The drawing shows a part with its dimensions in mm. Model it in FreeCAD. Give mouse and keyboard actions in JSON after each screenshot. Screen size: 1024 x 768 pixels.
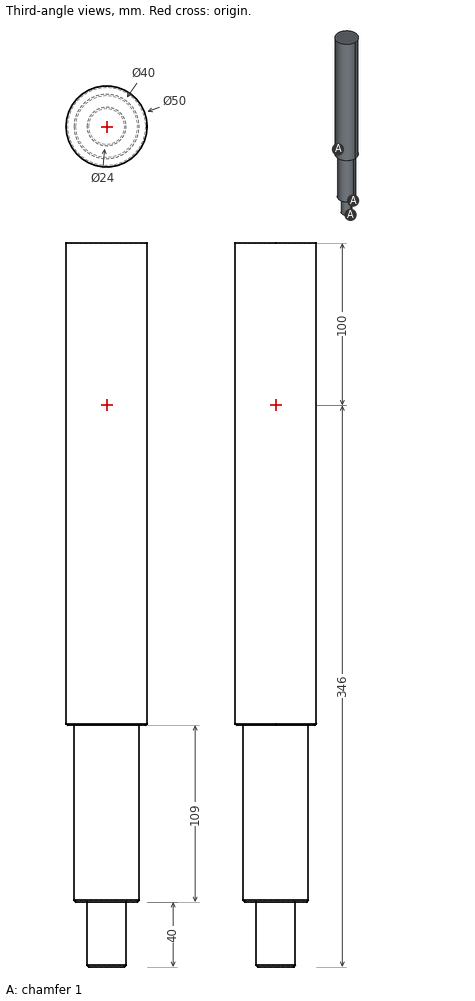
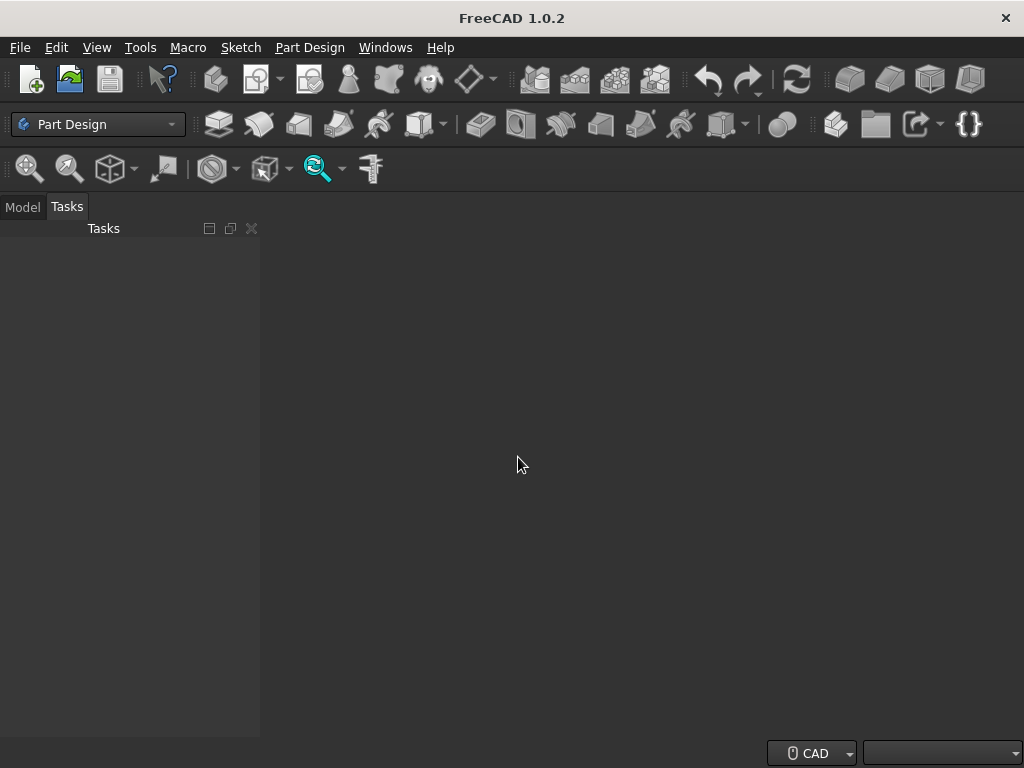
{"action": "left_click", "coordinate": [30, 80]}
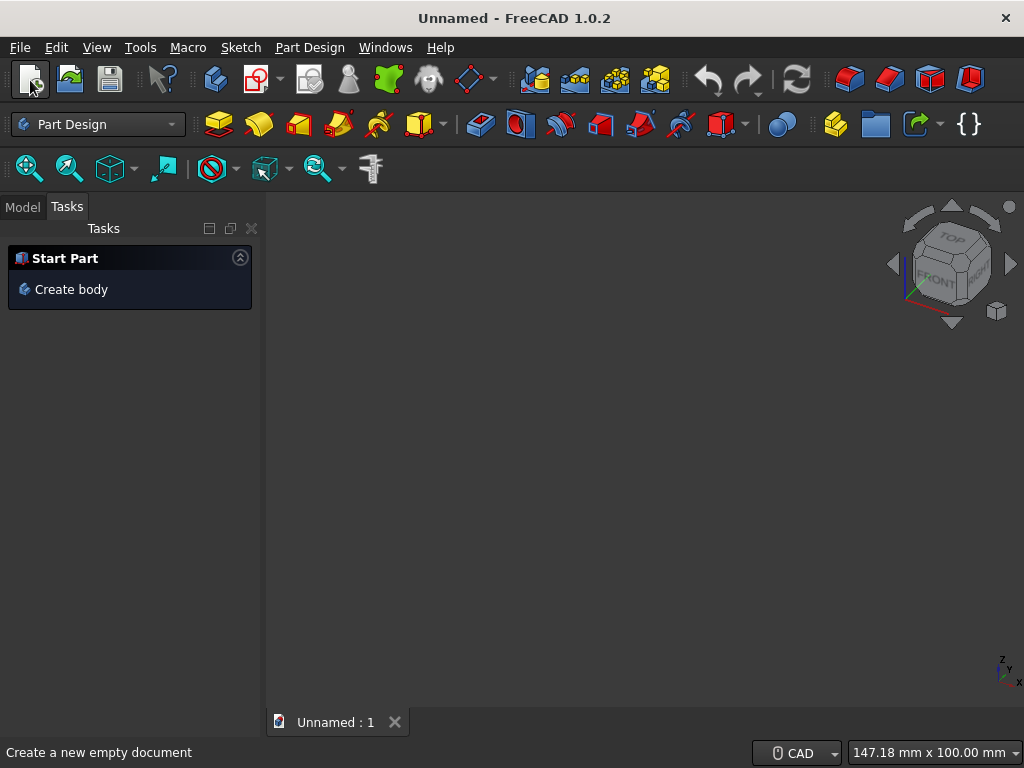
{"action": "left_click", "coordinate": [256, 80]}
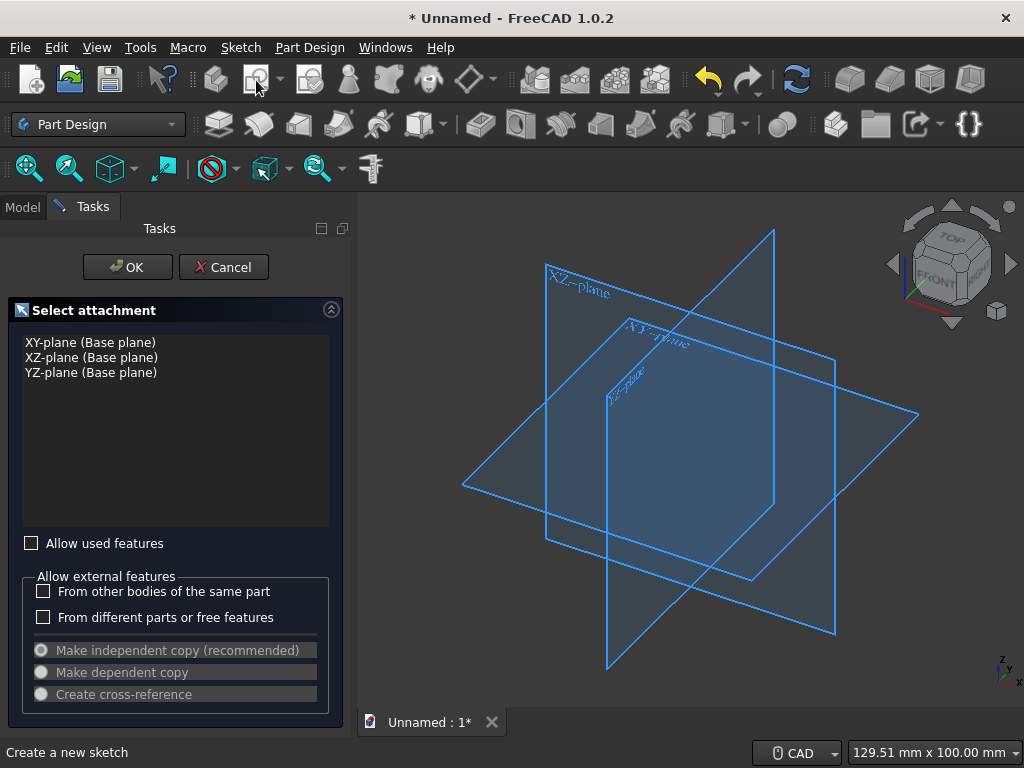
{"action": "left_click", "coordinate": [82, 342]}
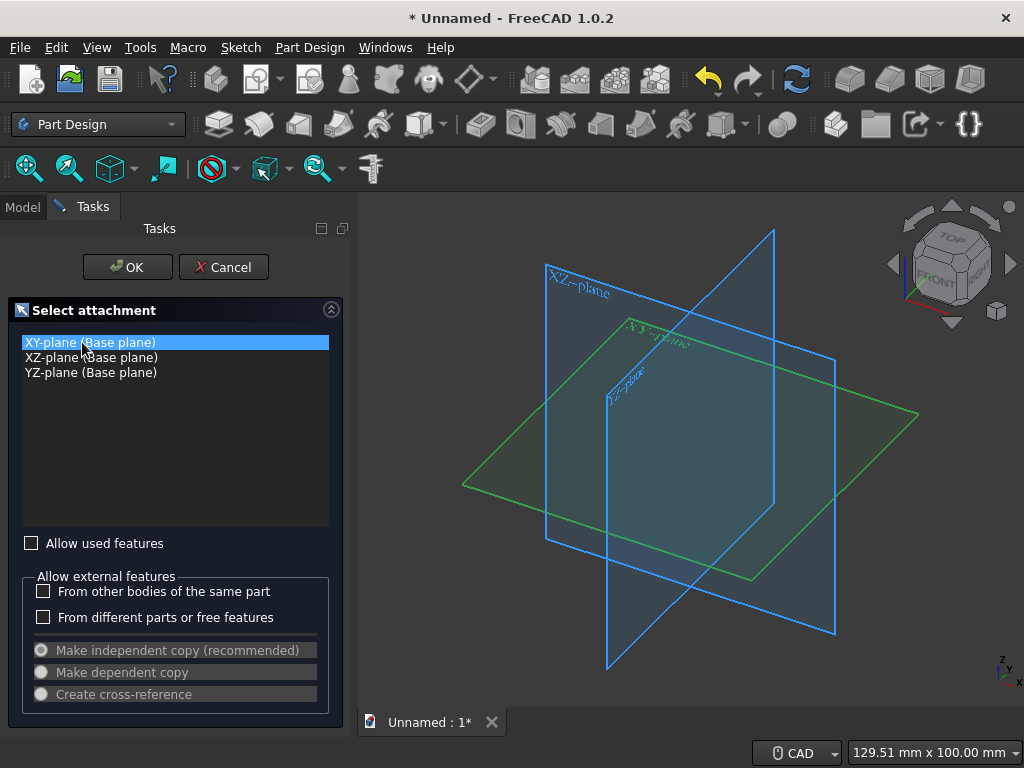
{"action": "left_click", "coordinate": [128, 267]}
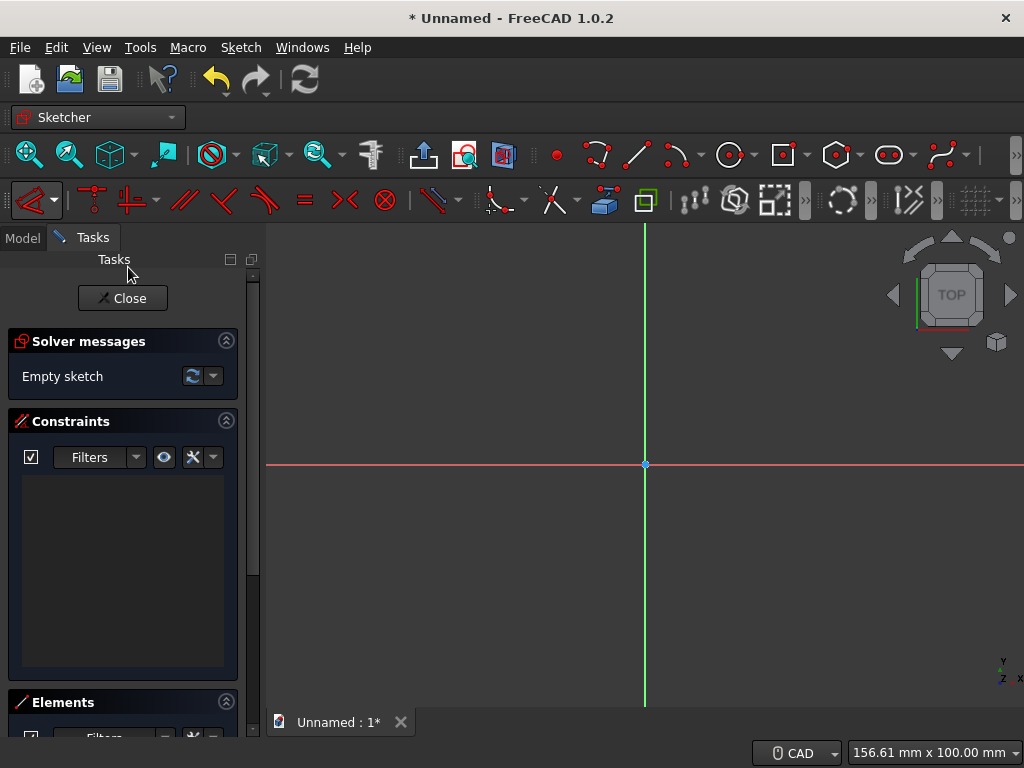
{"action": "left_click", "coordinate": [730, 156]}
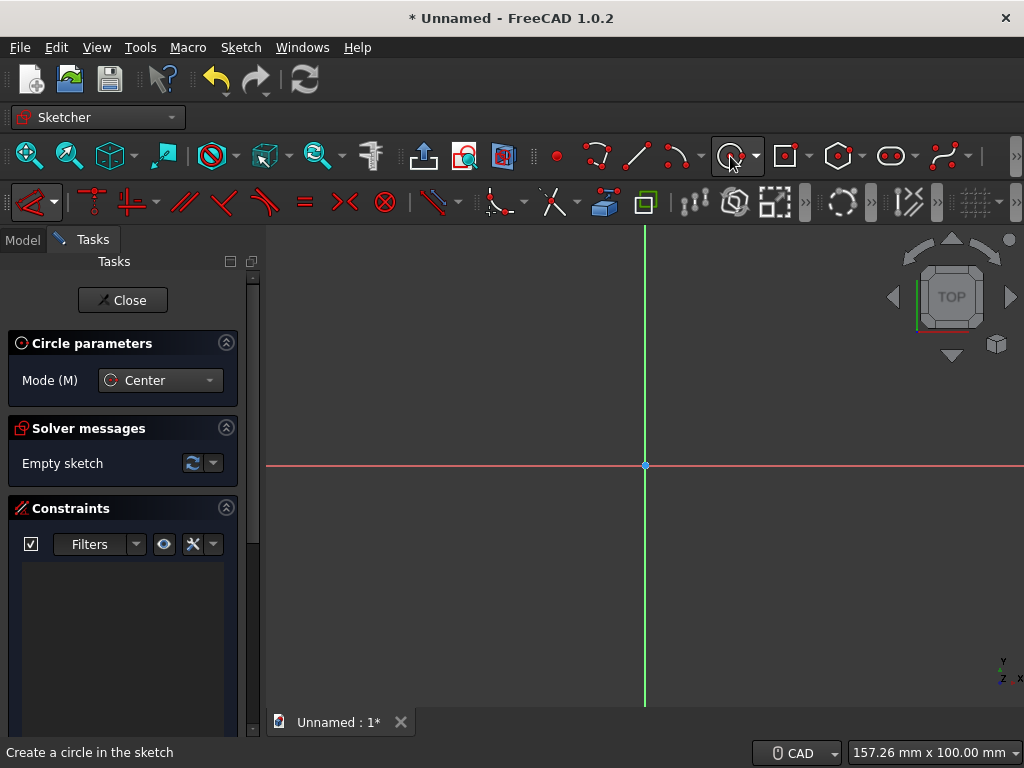
{"action": "left_click", "coordinate": [645, 466]}
{"action": "left_click", "coordinate": [730, 381]}
{"action": "key", "text": "Escape"}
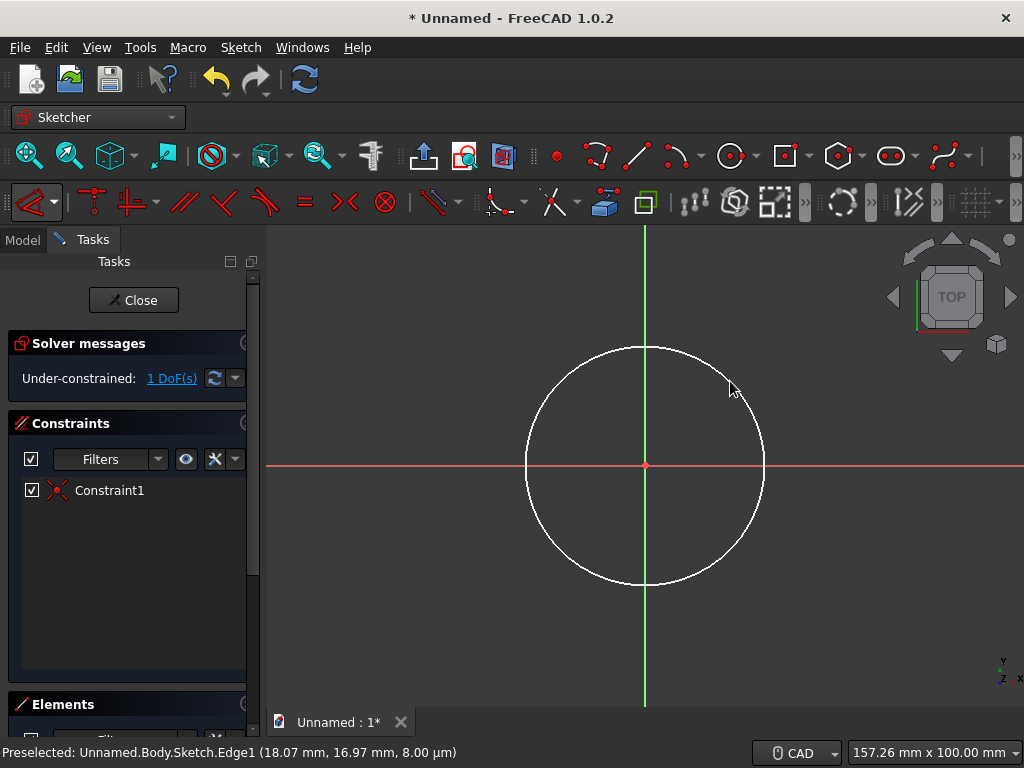
{"action": "left_click", "coordinate": [30, 202]}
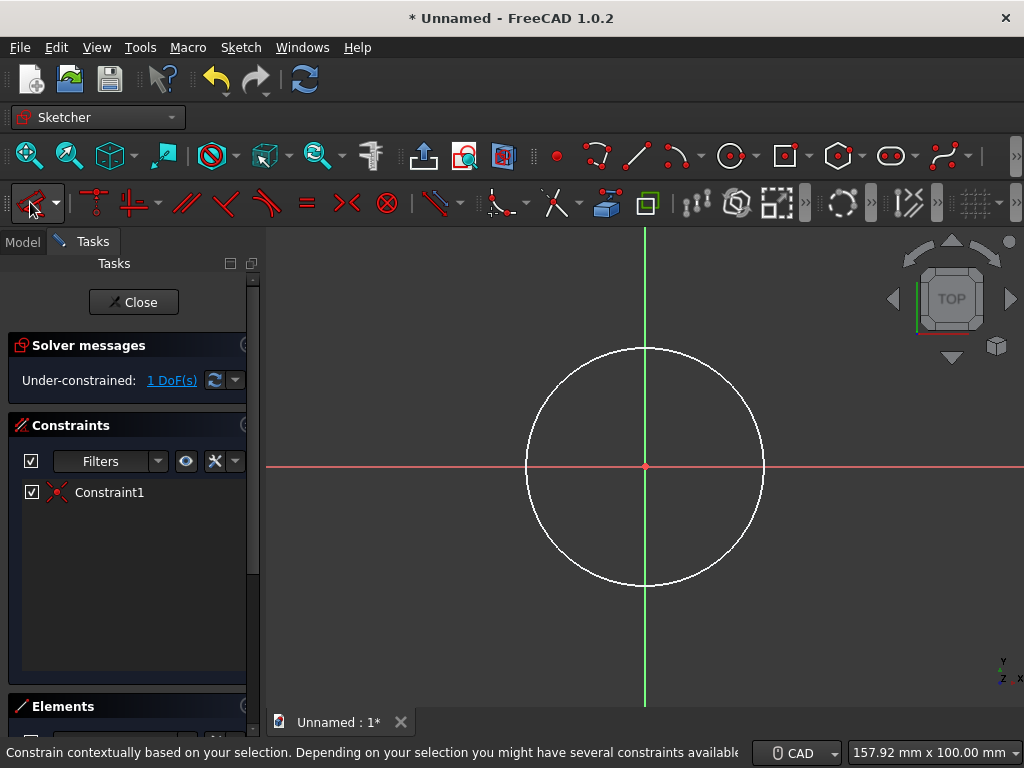
{"action": "left_click", "coordinate": [729, 383]}
{"action": "left_click", "coordinate": [752, 360]}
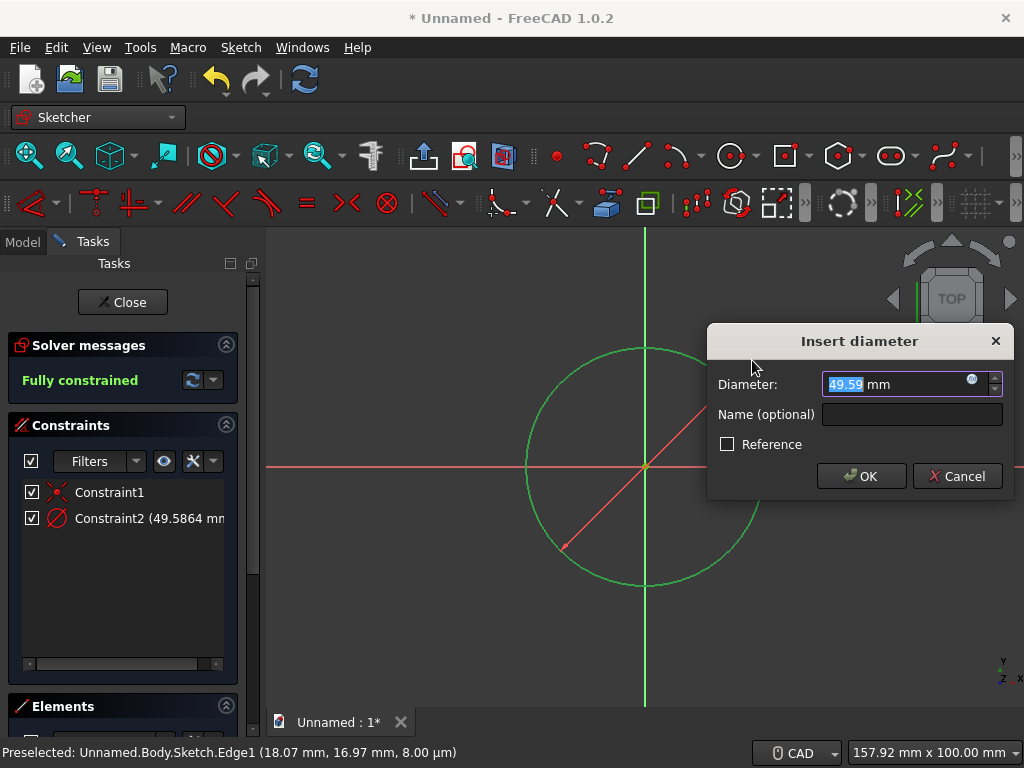
{"action": "type", "text": "50"}
{"action": "key", "text": "Return"}
{"action": "key", "text": "Escape"}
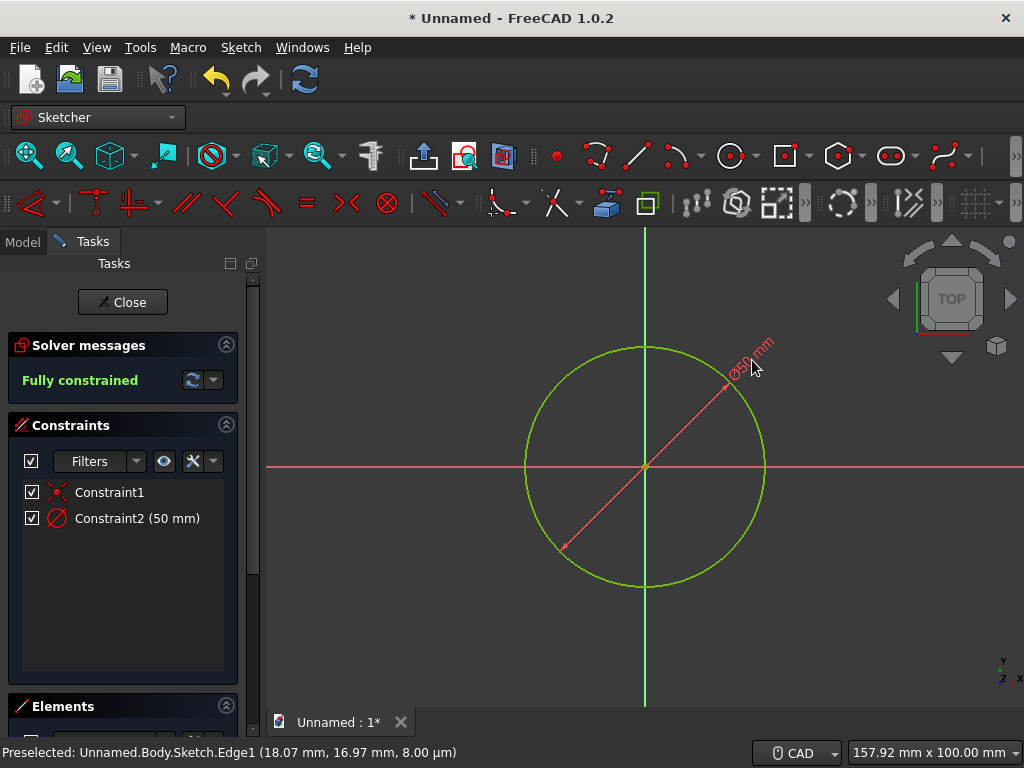
{"action": "left_click", "coordinate": [123, 302]}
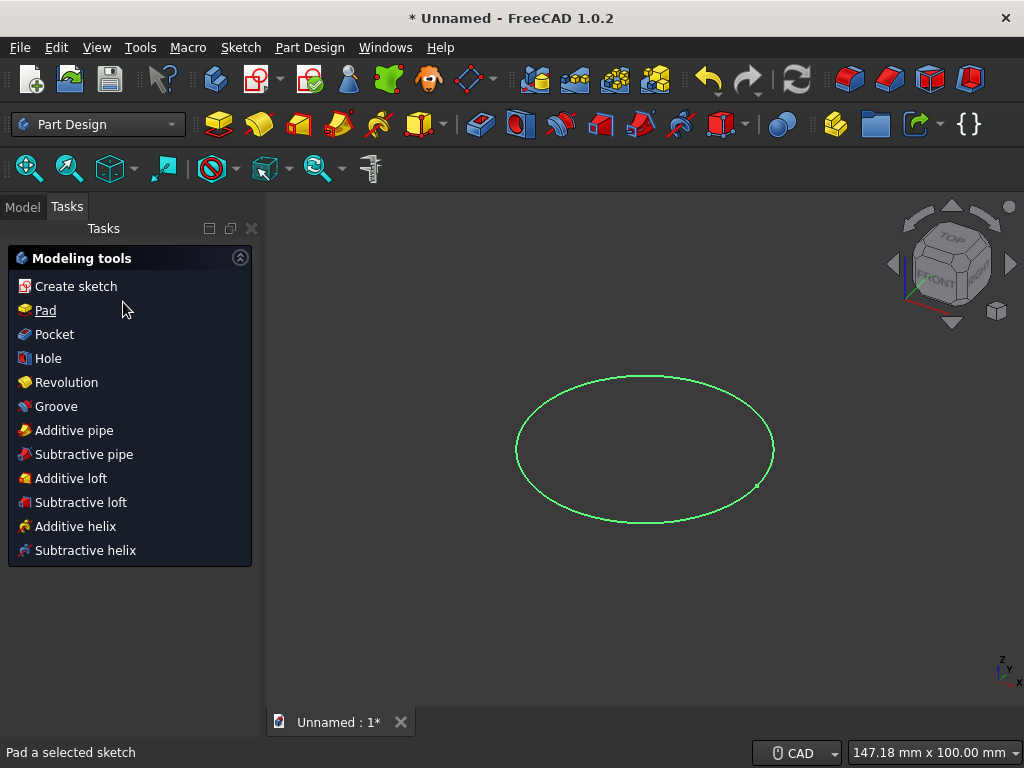
{"action": "left_click", "coordinate": [220, 124]}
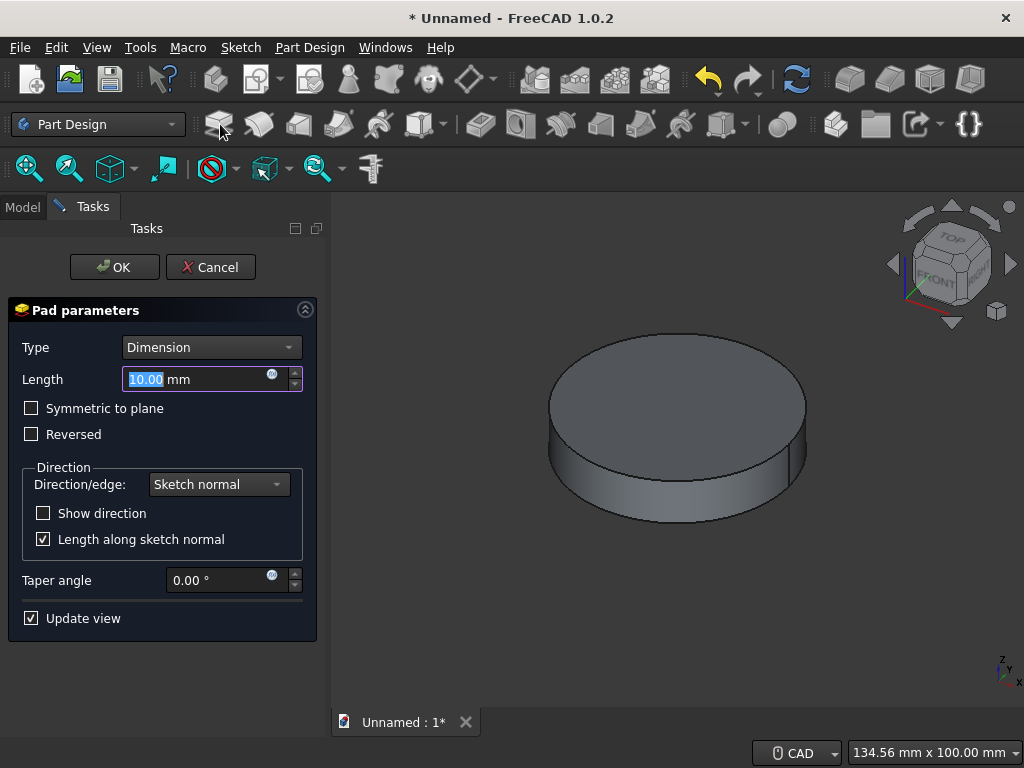
{"action": "left_click", "coordinate": [212, 348]}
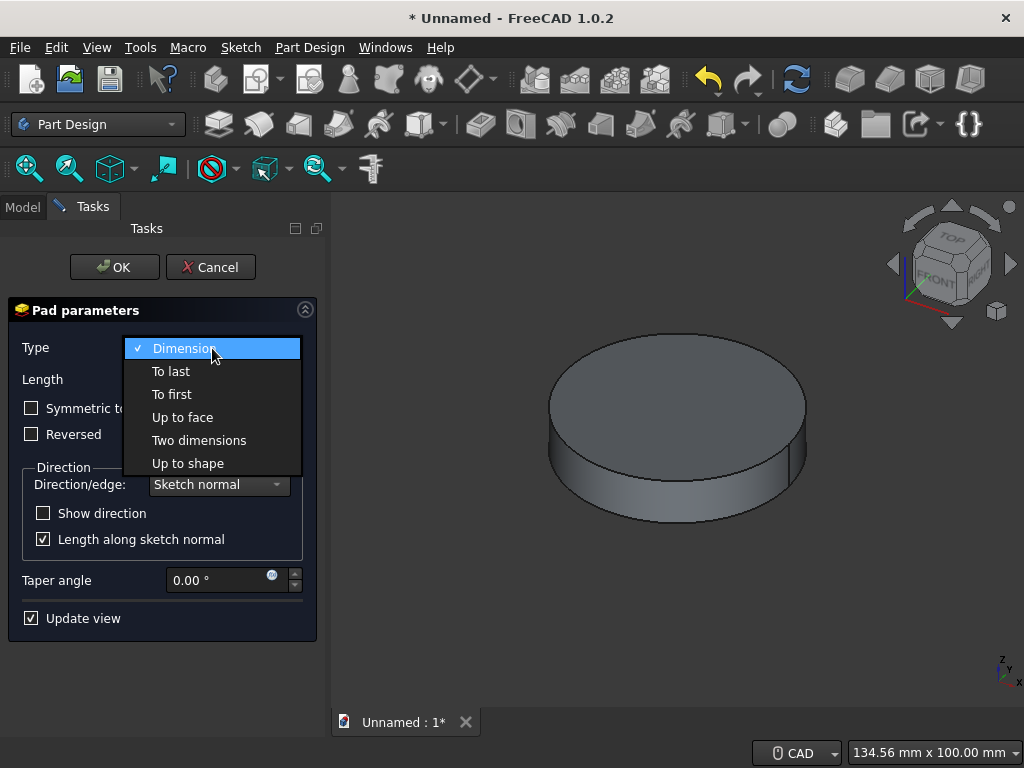
{"action": "left_click", "coordinate": [212, 440]}